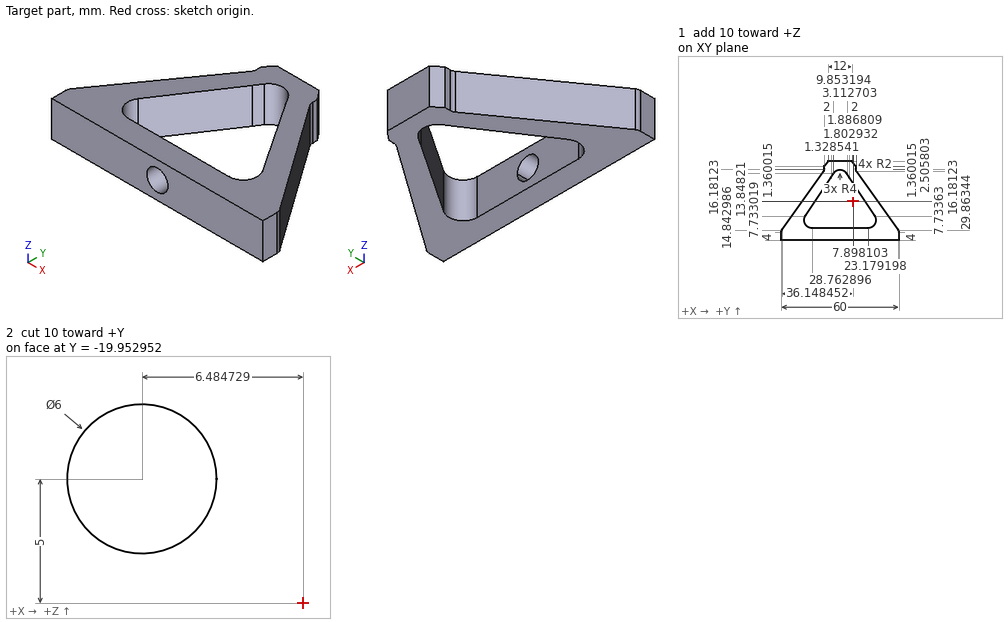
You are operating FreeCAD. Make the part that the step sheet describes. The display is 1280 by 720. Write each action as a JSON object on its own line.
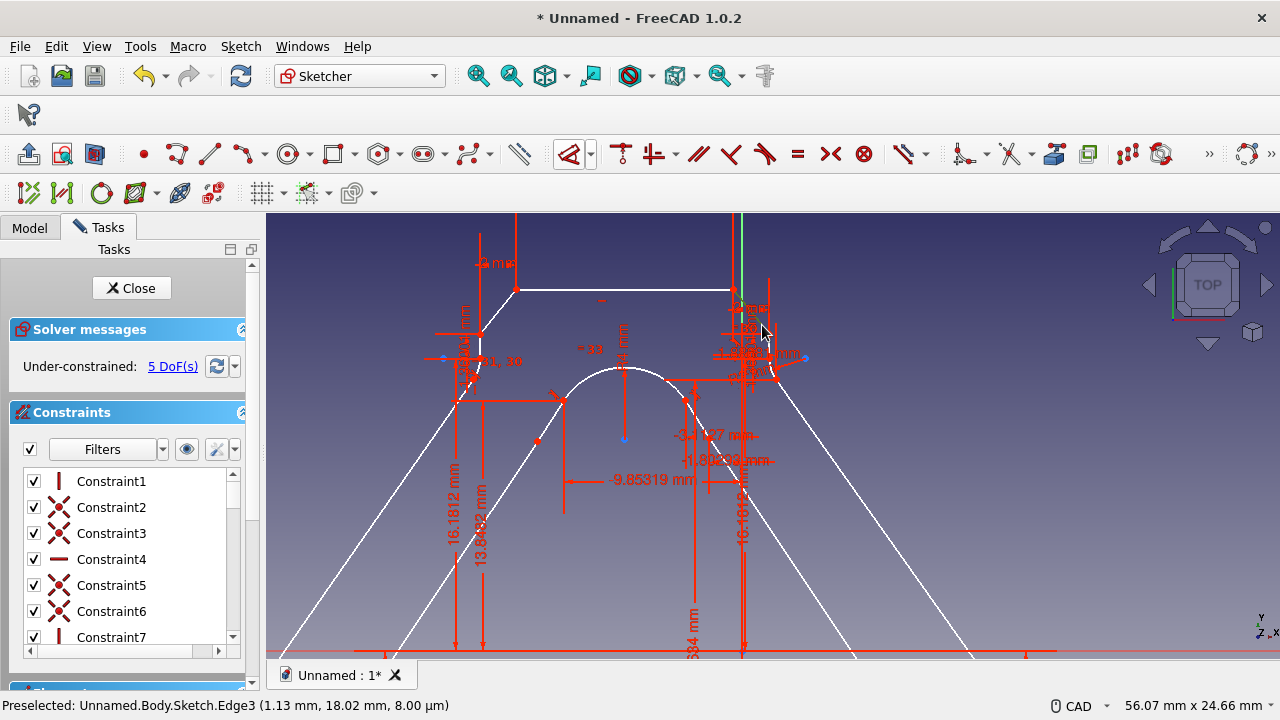
{"action": "left_click", "coordinate": [590, 154]}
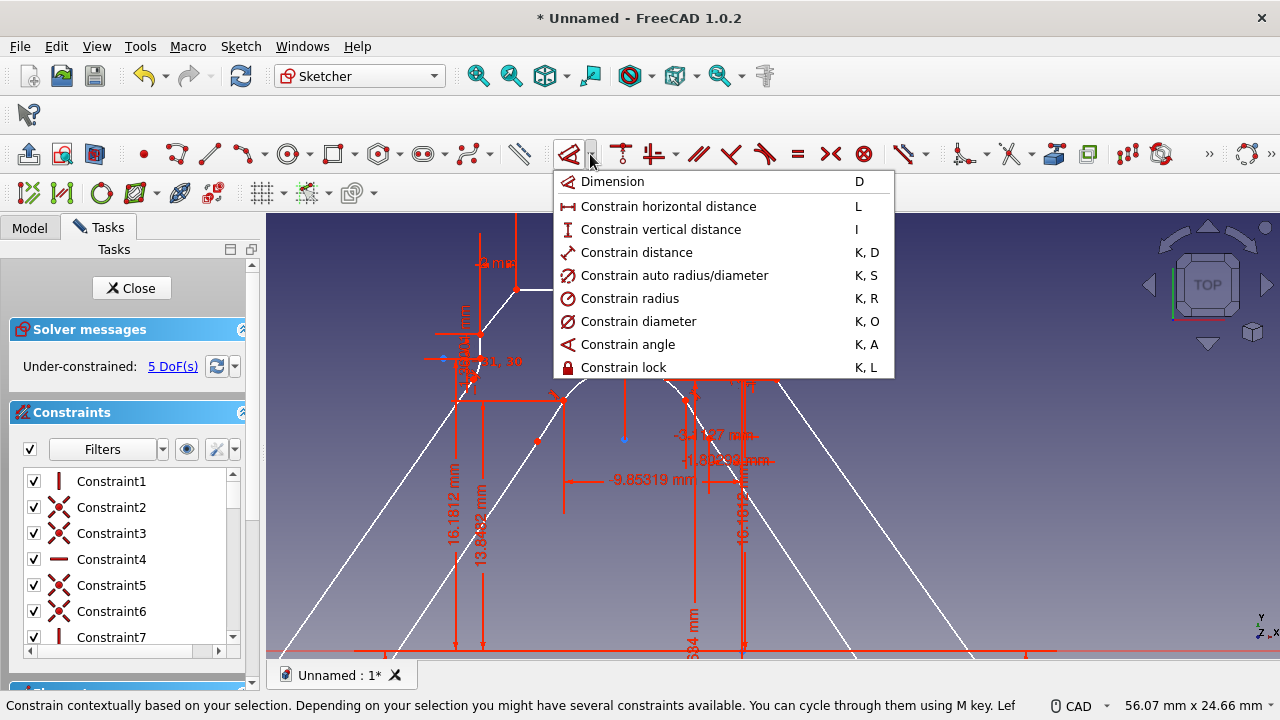
{"action": "left_click", "coordinate": [724, 230]}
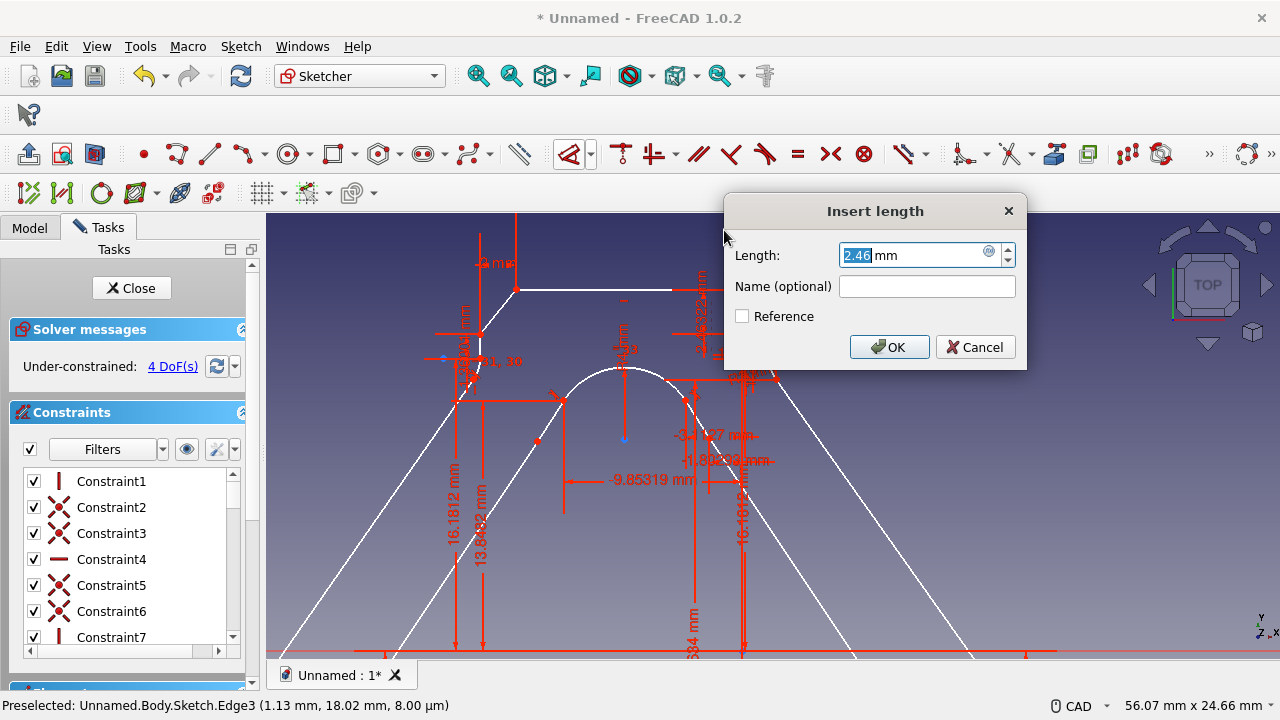
{"action": "type", "text": "2.505803"}
{"action": "key", "text": "Return"}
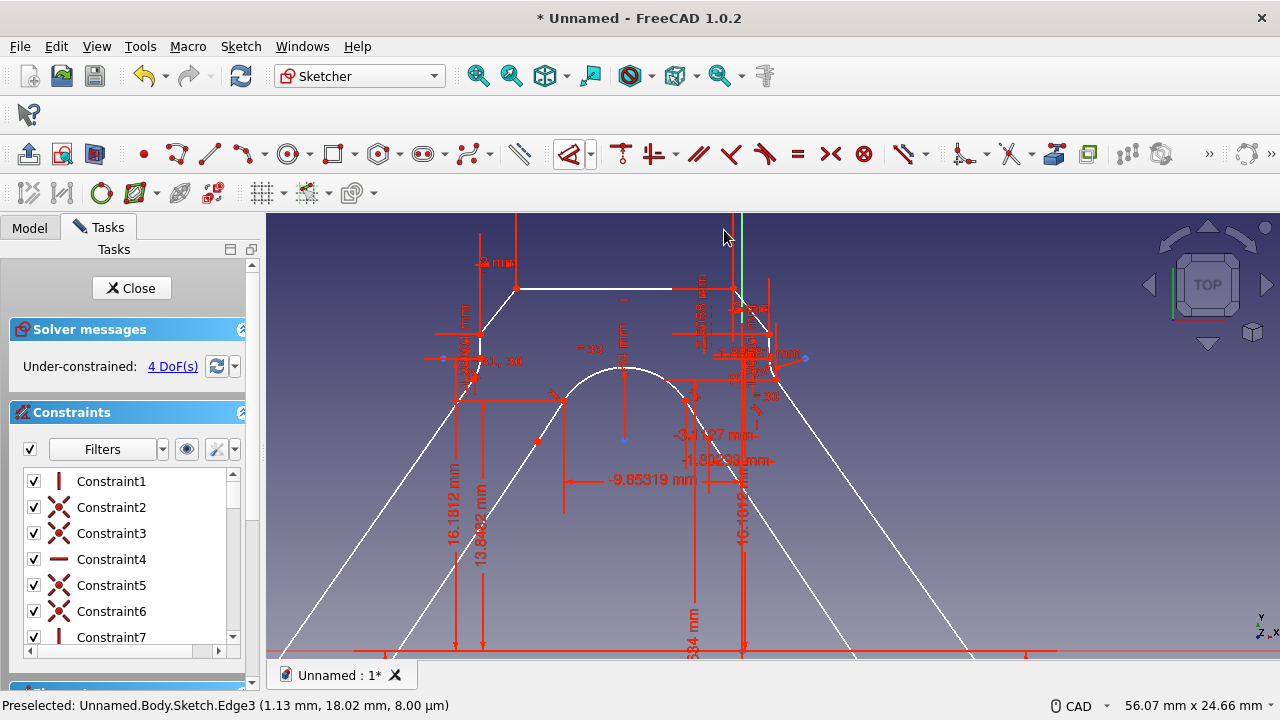
{"action": "scroll", "coordinate": [546, 429], "scroll_direction": "up", "scroll_amount": 3}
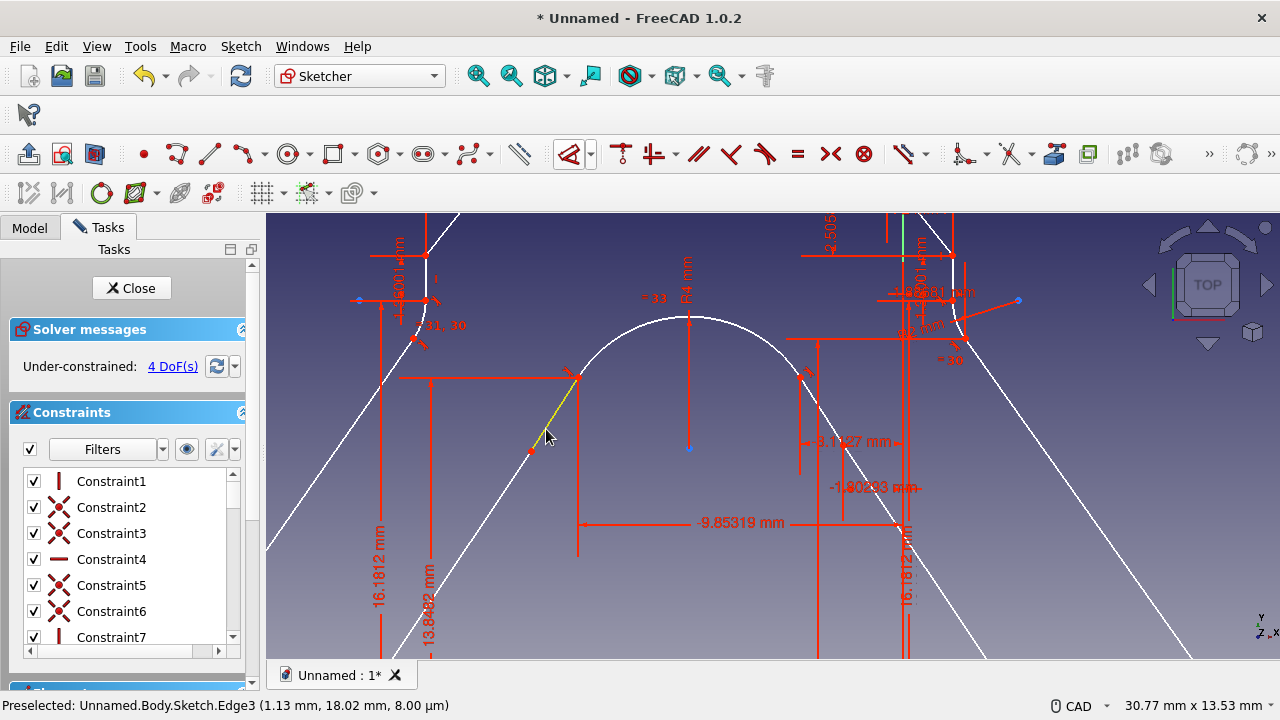
{"action": "left_click", "coordinate": [545, 429]}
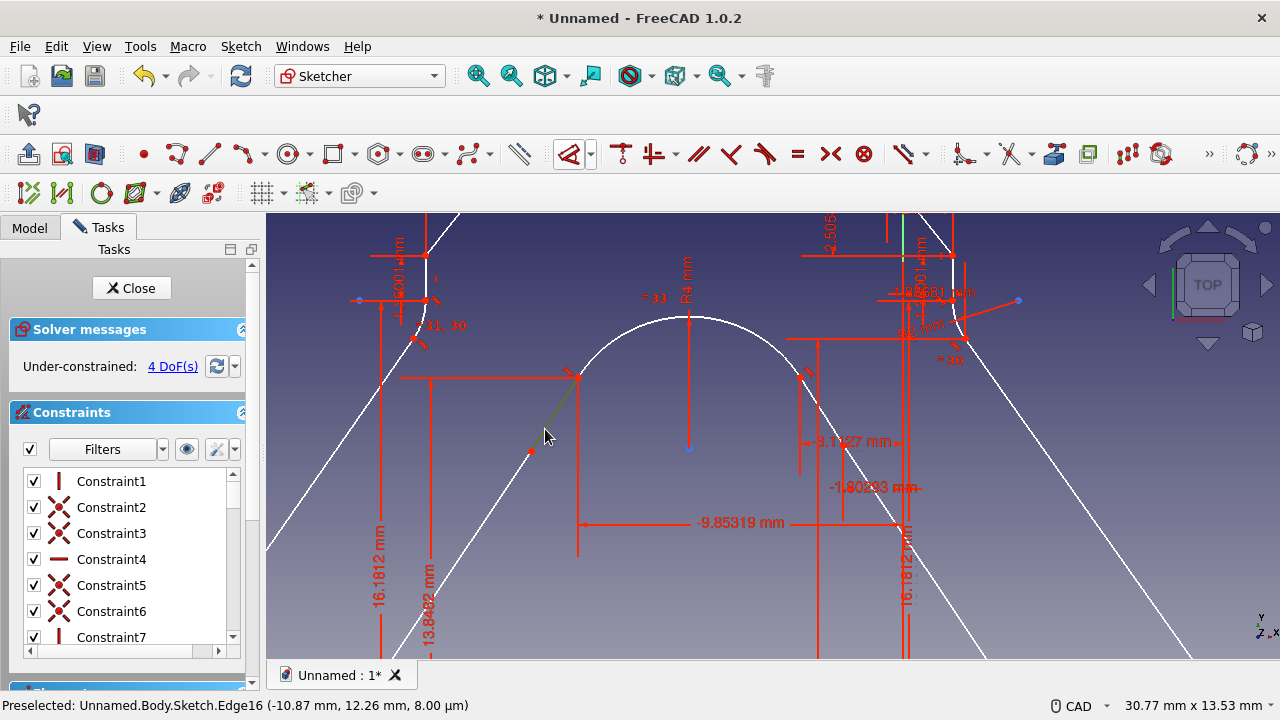
{"action": "key", "text": "l"}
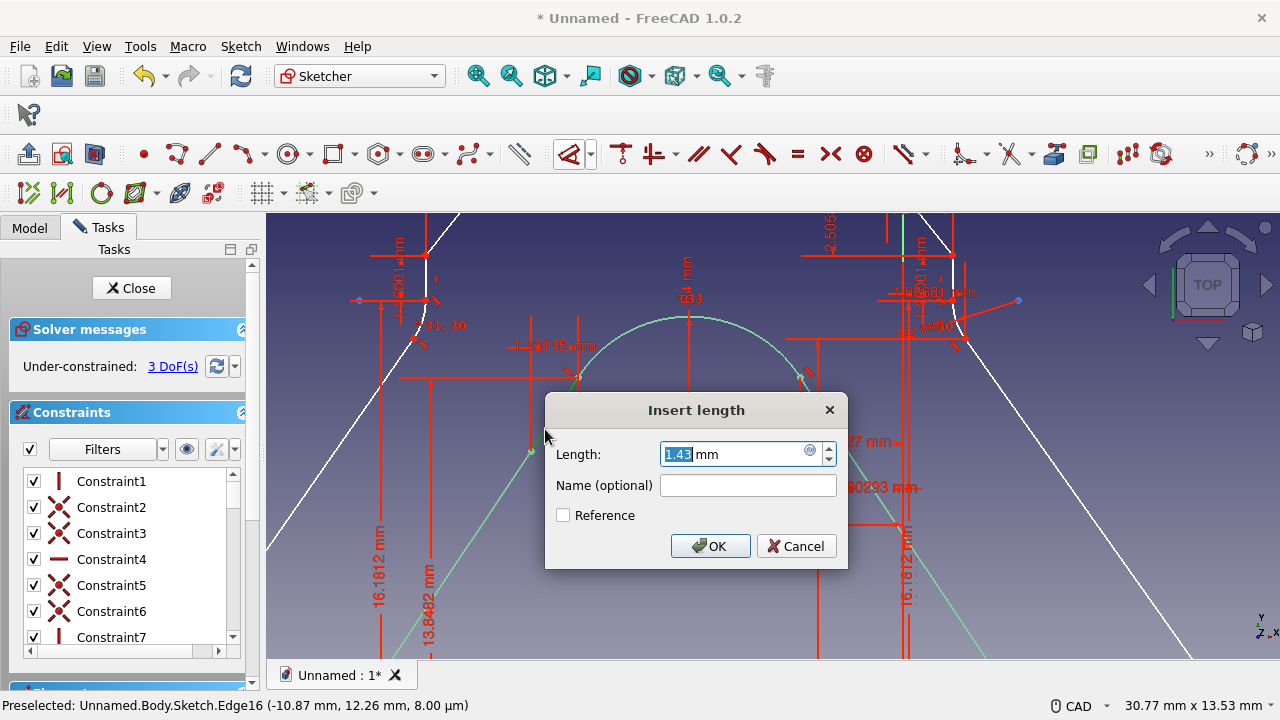
{"action": "type", "text": "1.328541"}
{"action": "key", "text": "Return"}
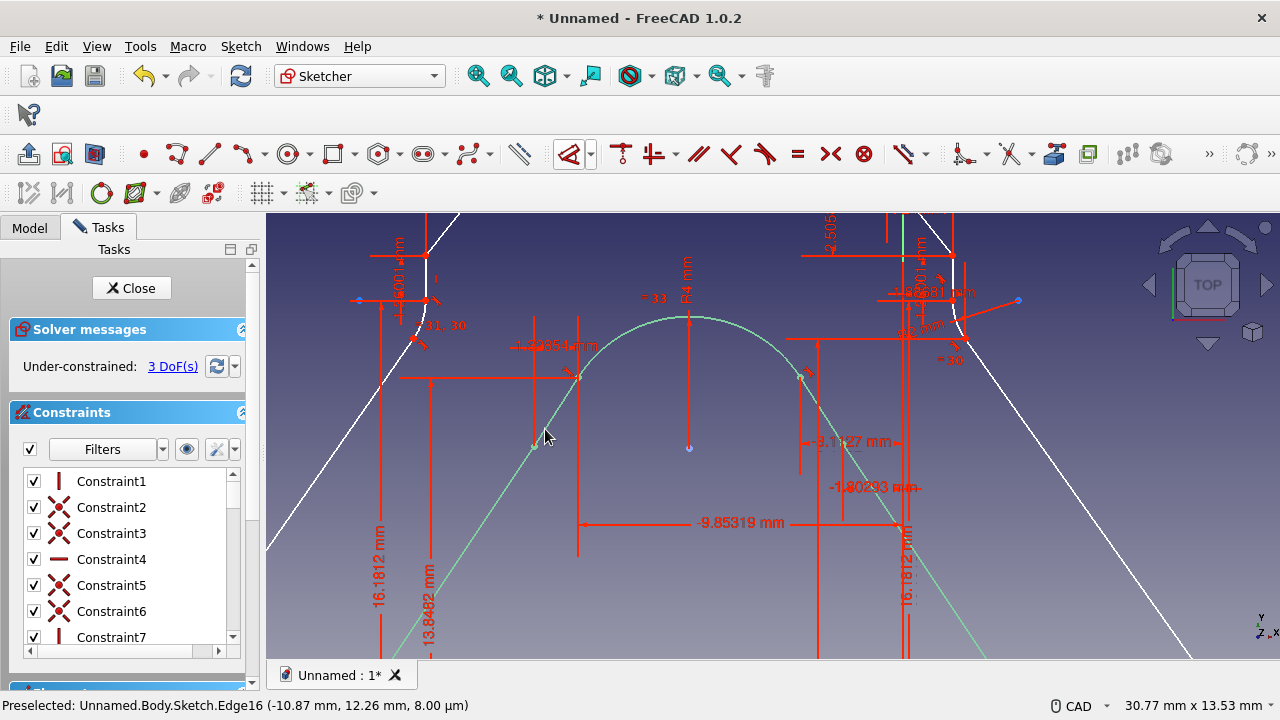
{"action": "scroll", "coordinate": [708, 336], "scroll_direction": "down", "scroll_amount": 8}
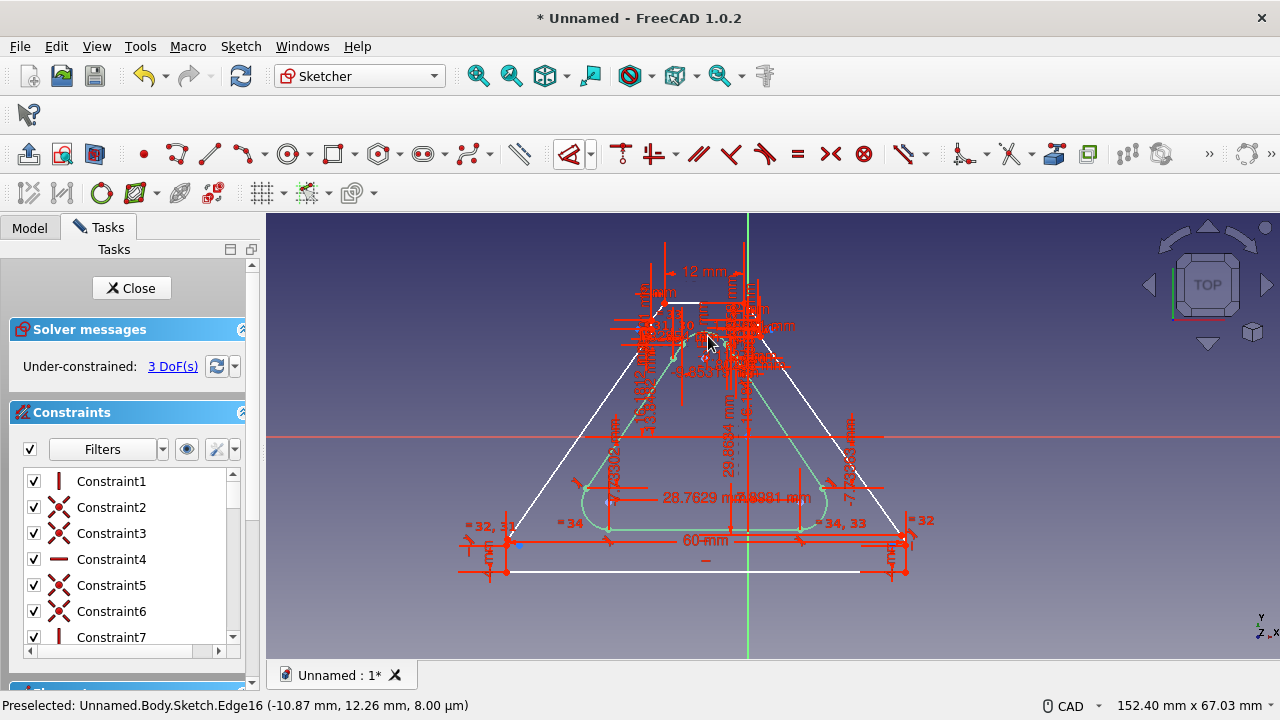
{"action": "left_click", "coordinate": [901, 535]}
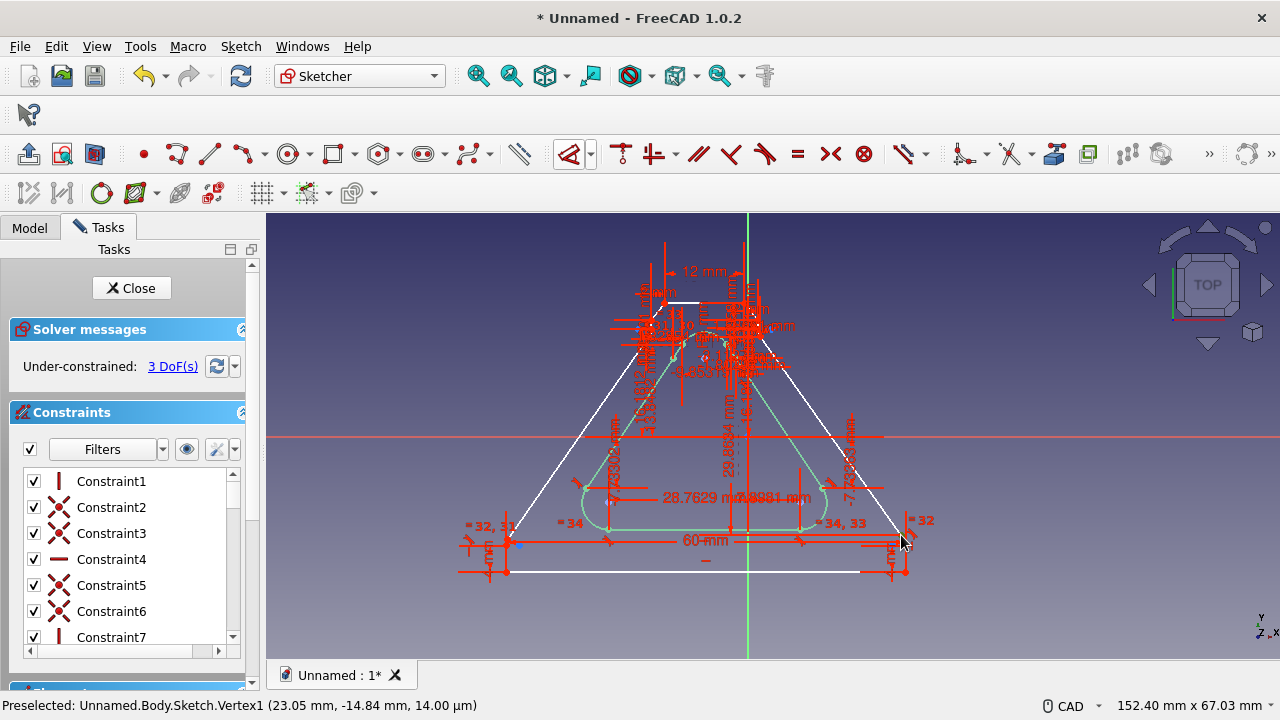
{"action": "key", "text": "l"}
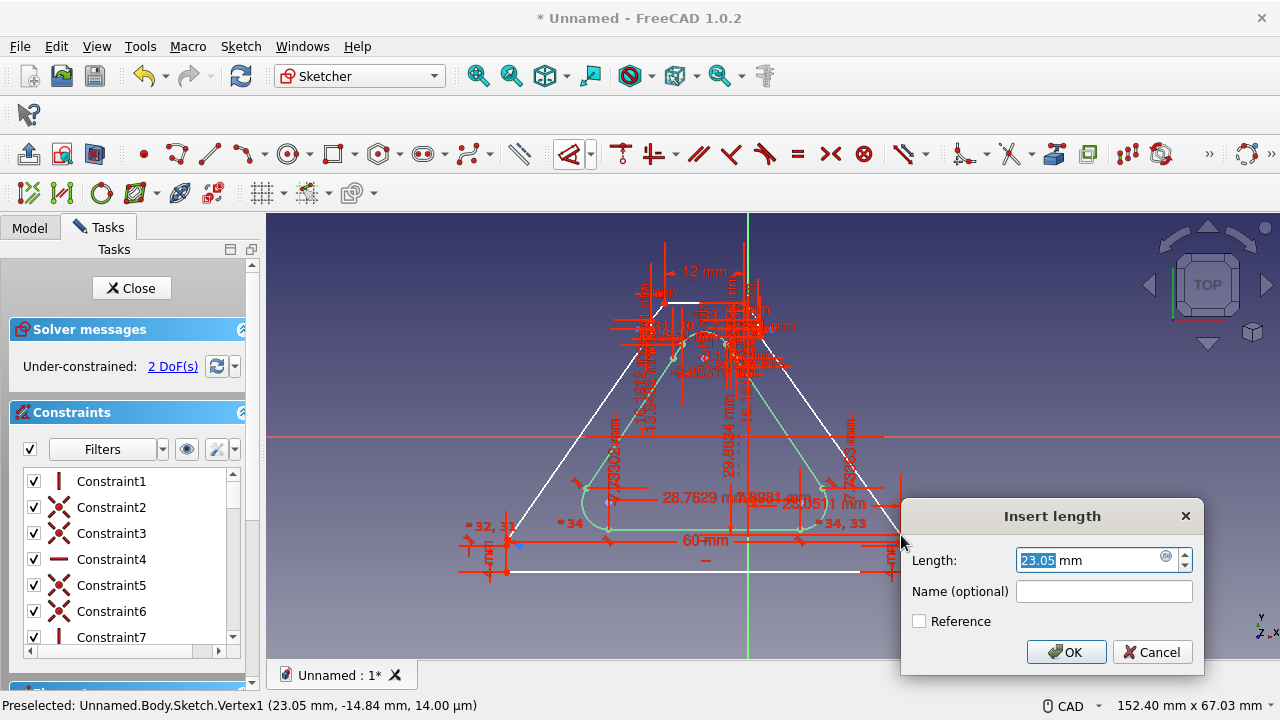
{"action": "type", "text": "23.179198"}
{"action": "key", "text": "Return"}